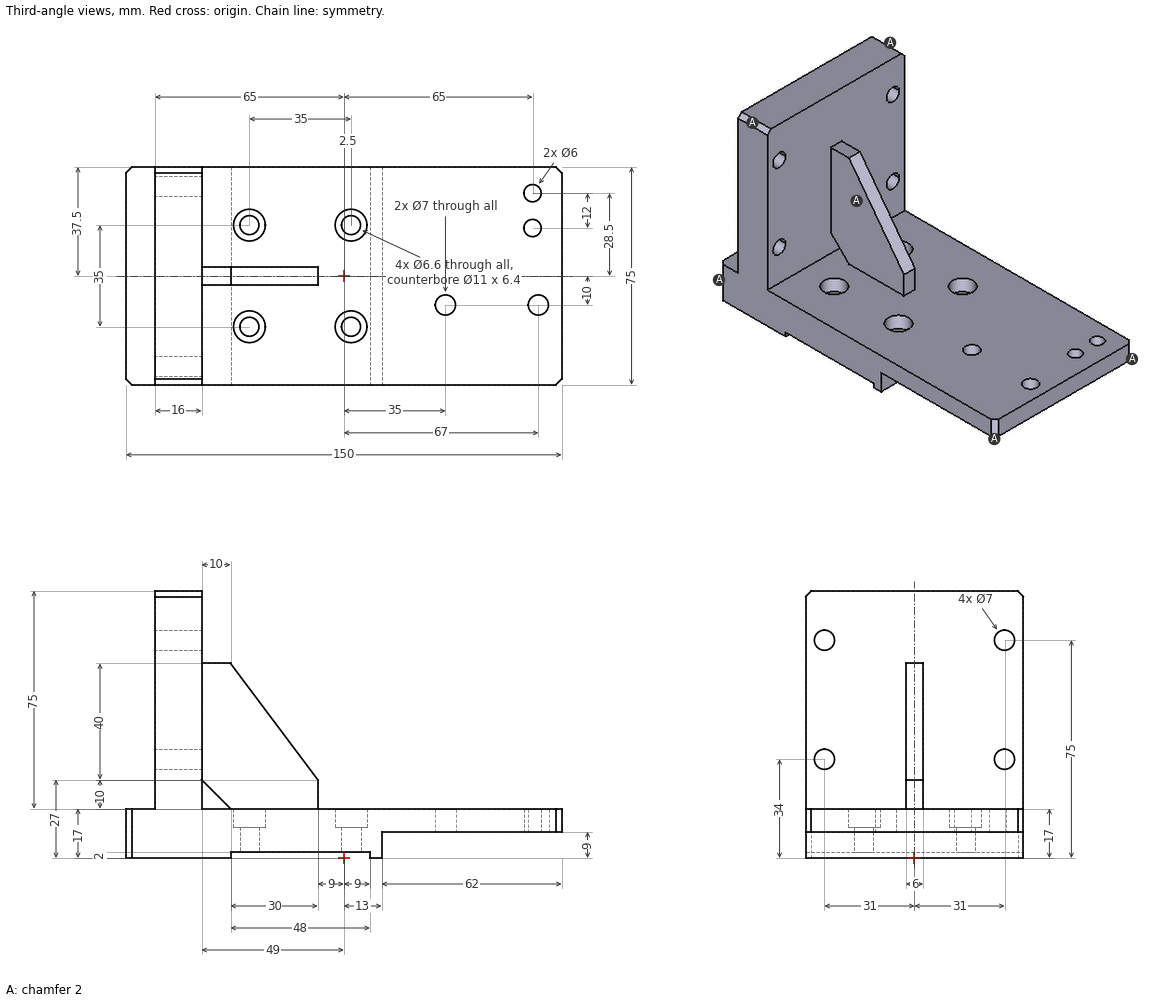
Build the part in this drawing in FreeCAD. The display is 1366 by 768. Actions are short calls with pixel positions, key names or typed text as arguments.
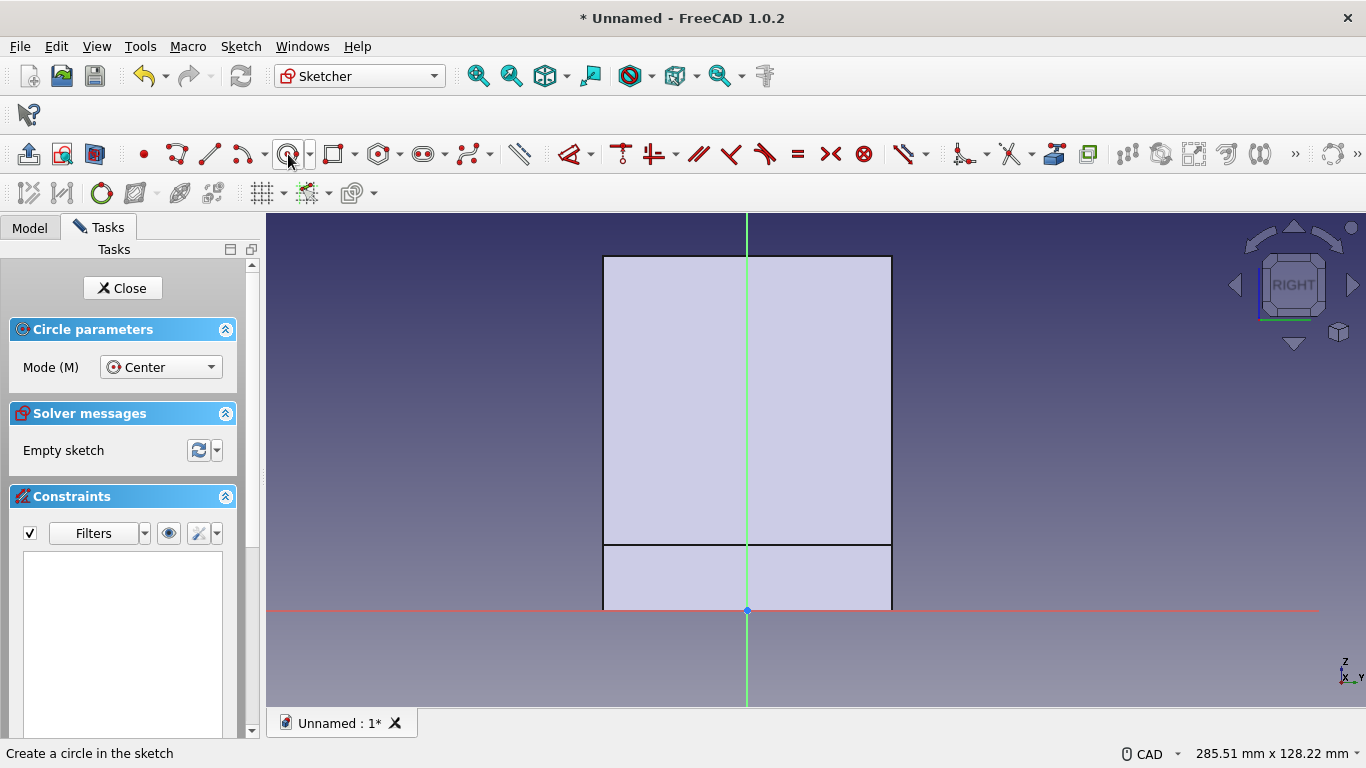
scroll(867, 322, up, 3)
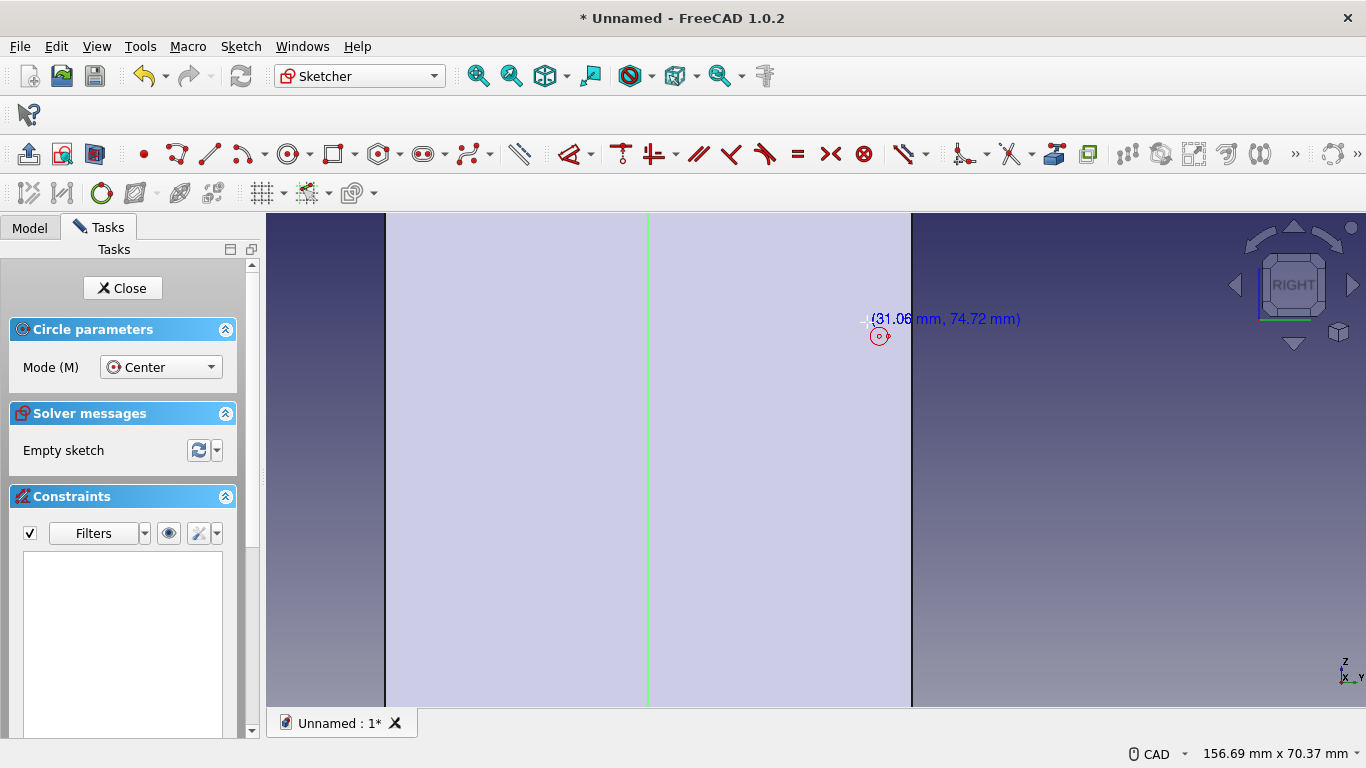
click(866, 322)
move(883, 304)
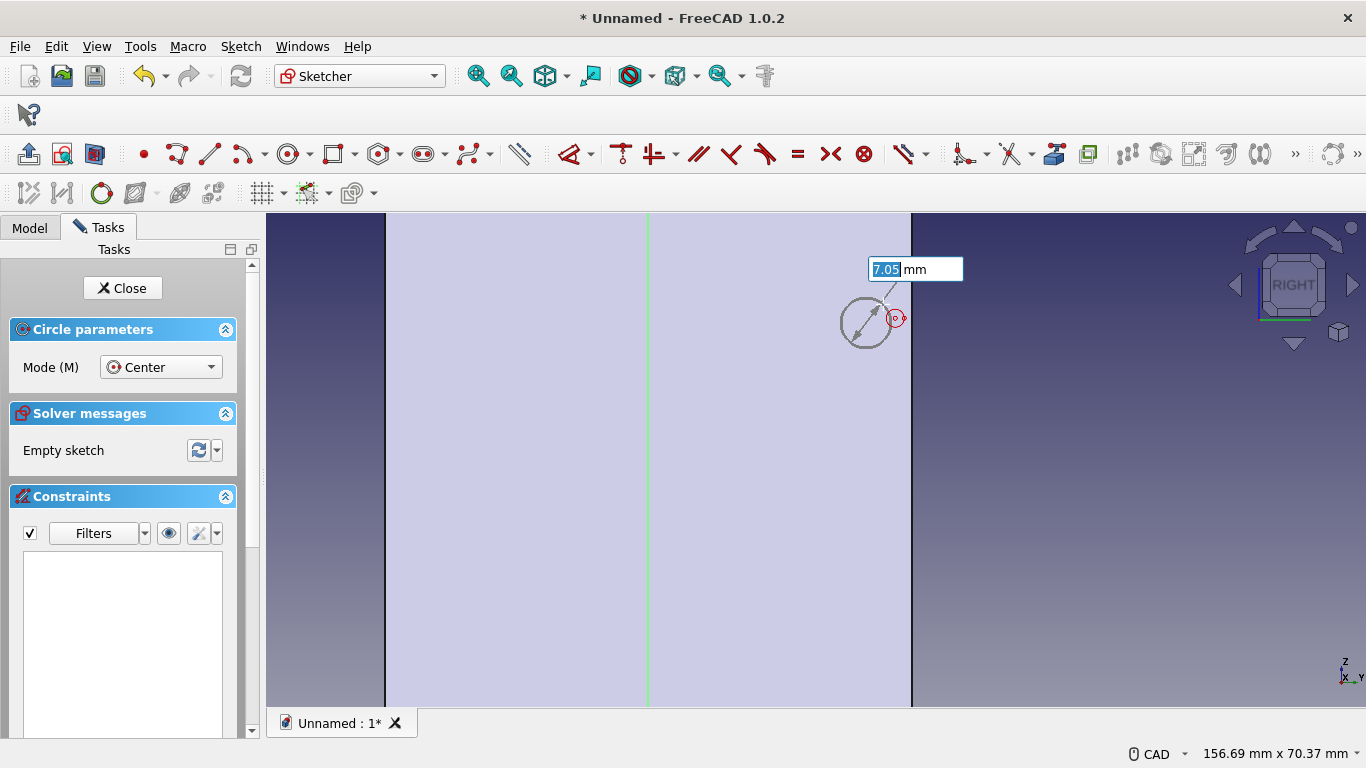
text(7)
key(Return)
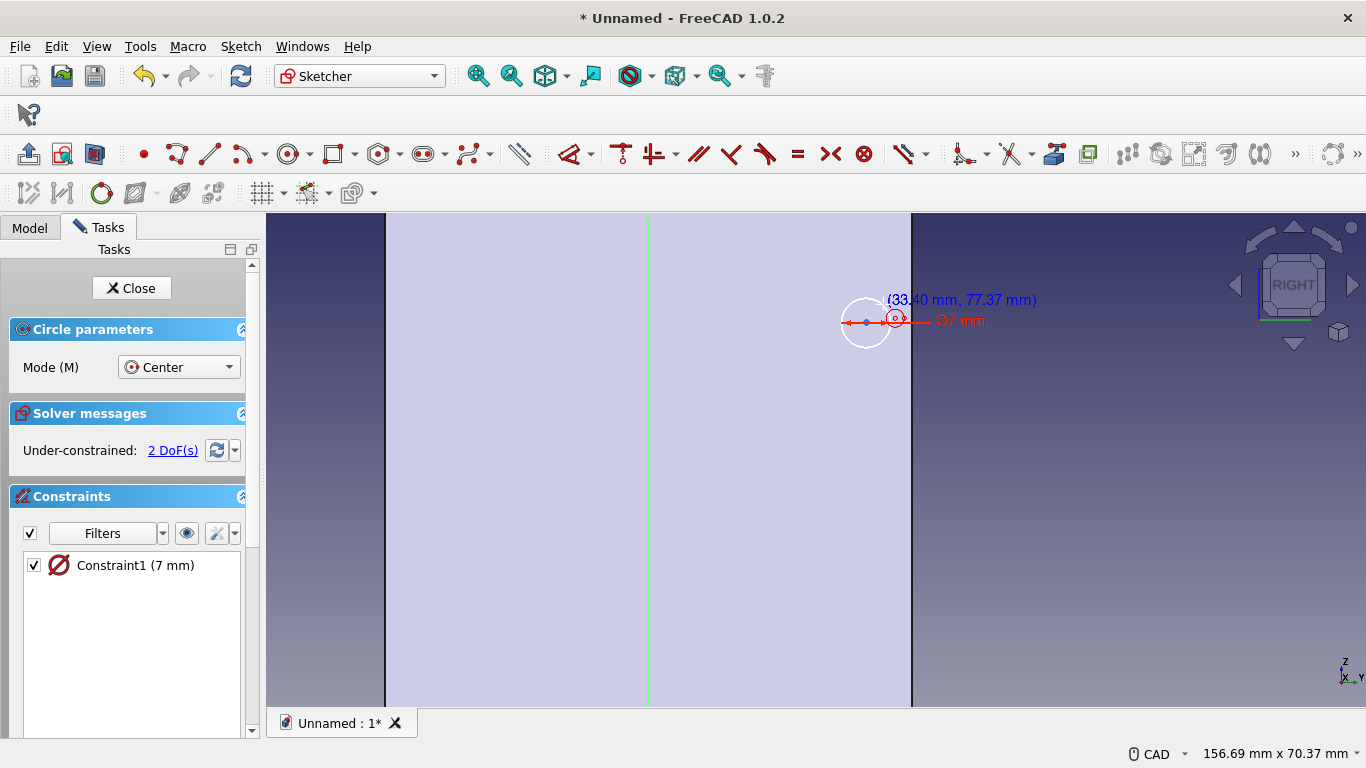
click(431, 322)
move(448, 304)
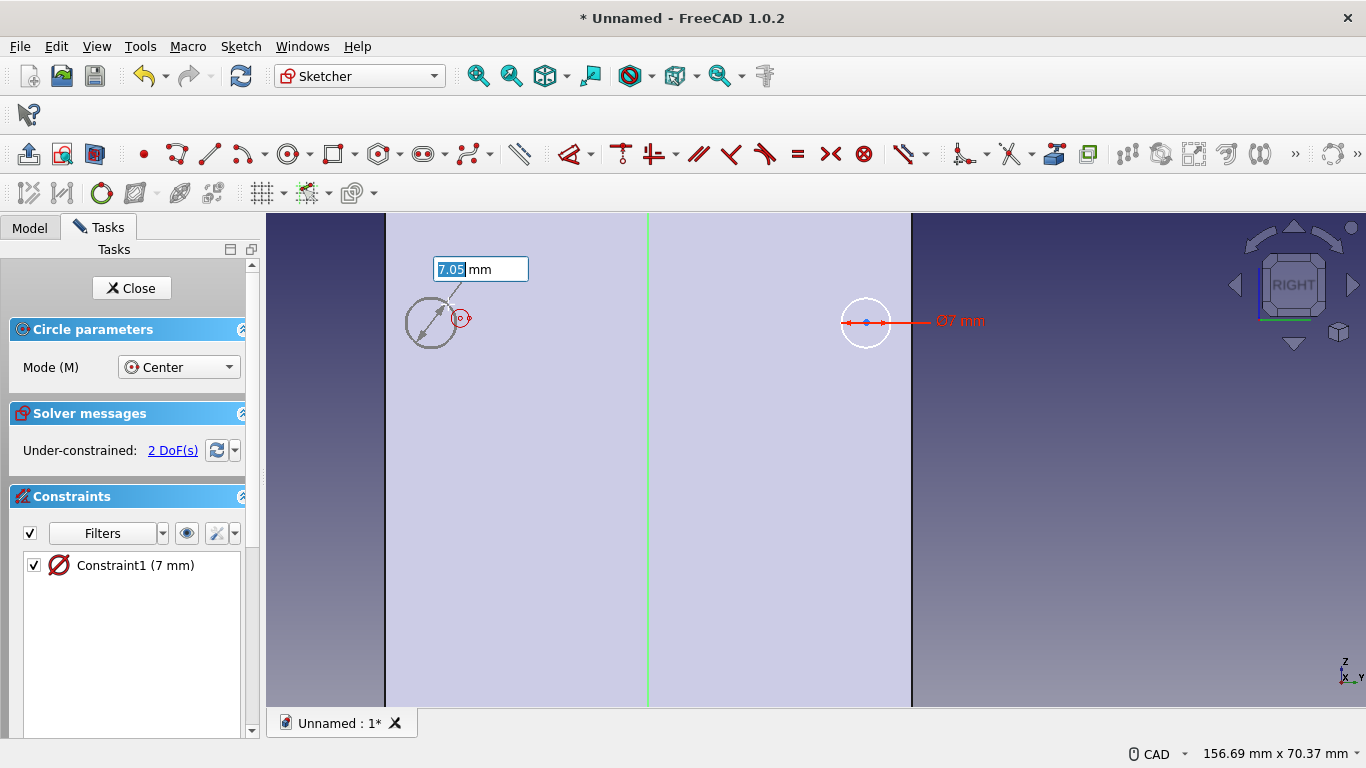
text(7)
key(Return)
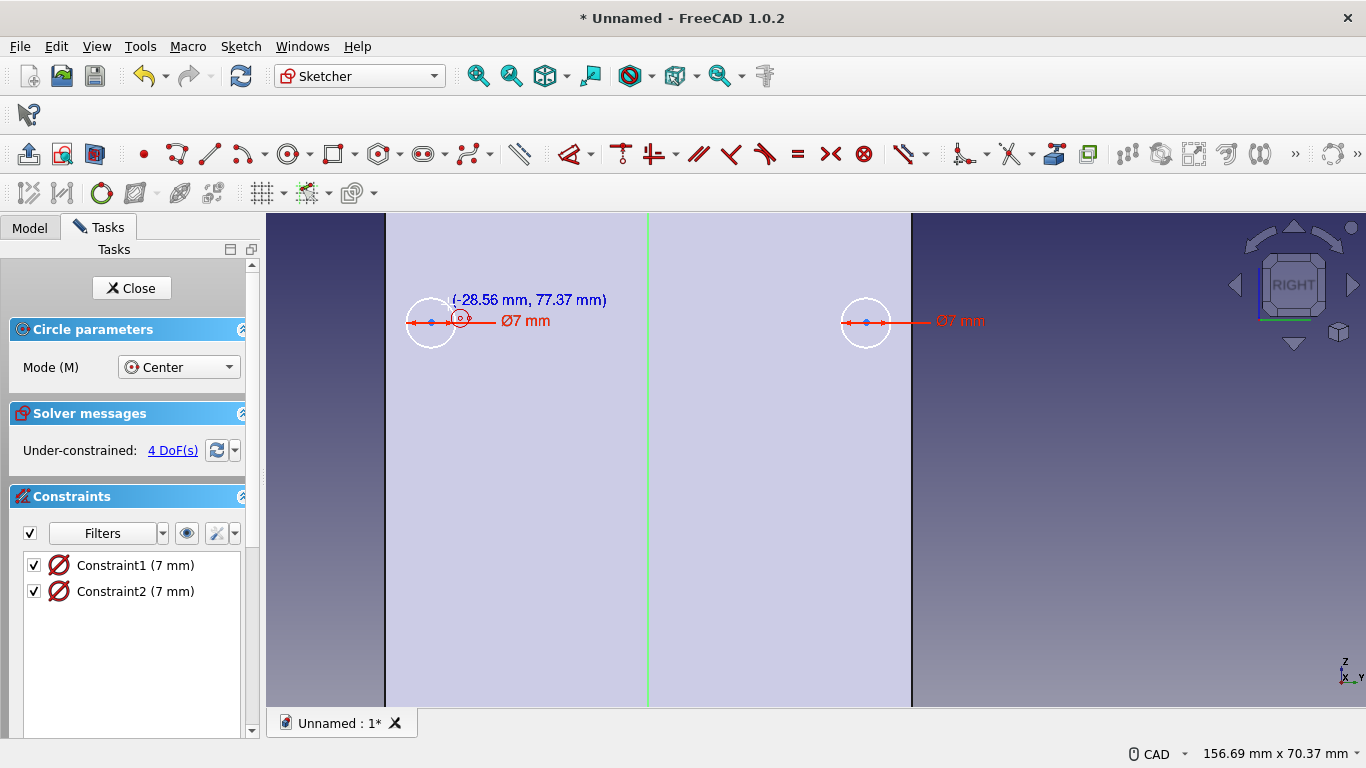
click(431, 609)
move(448, 592)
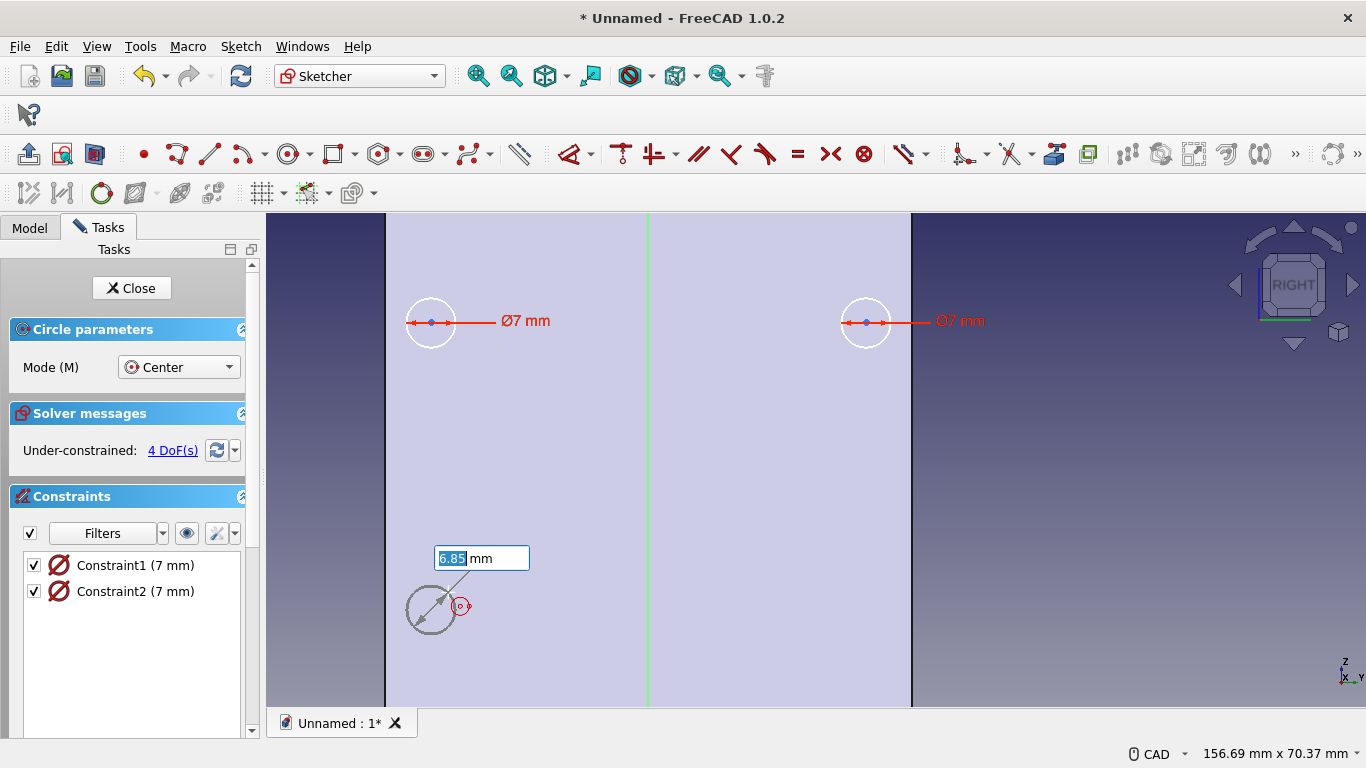
text(7)
key(Return)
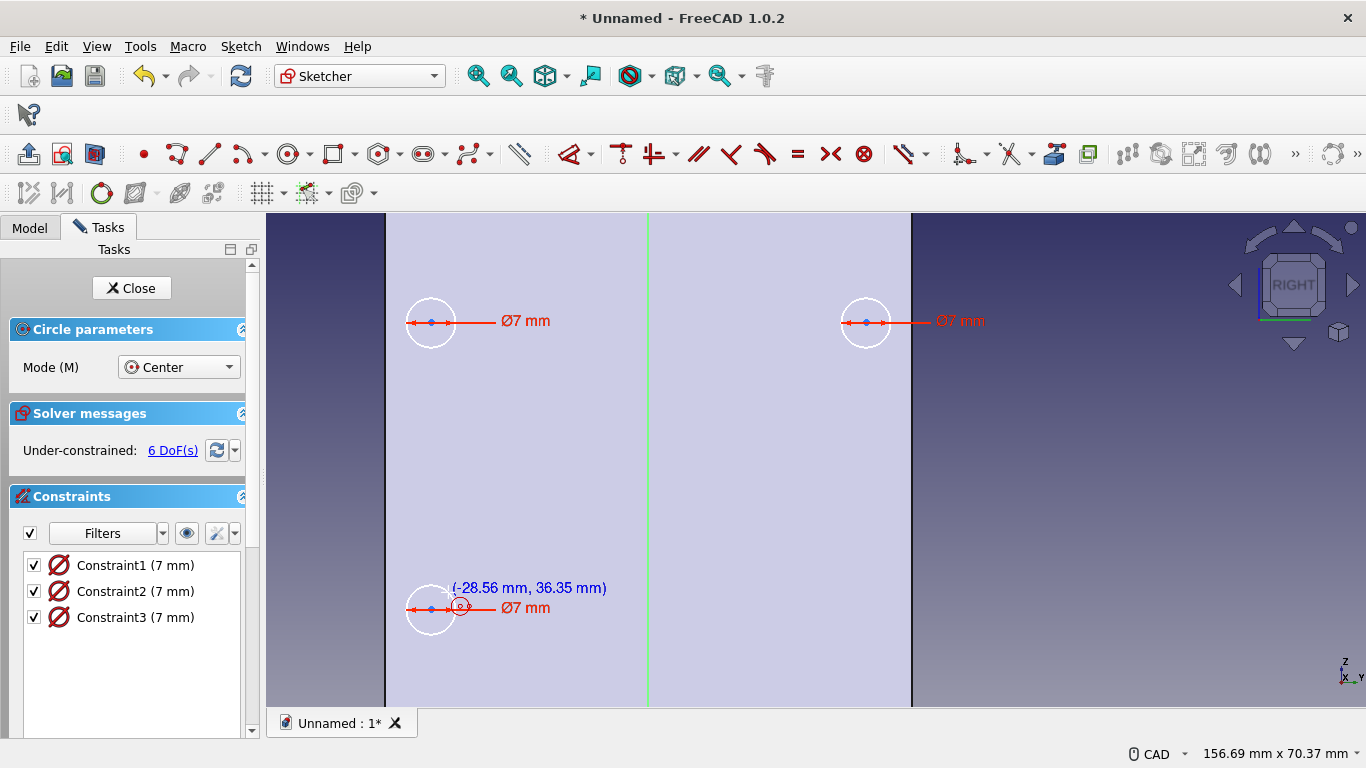
click(866, 609)
move(883, 592)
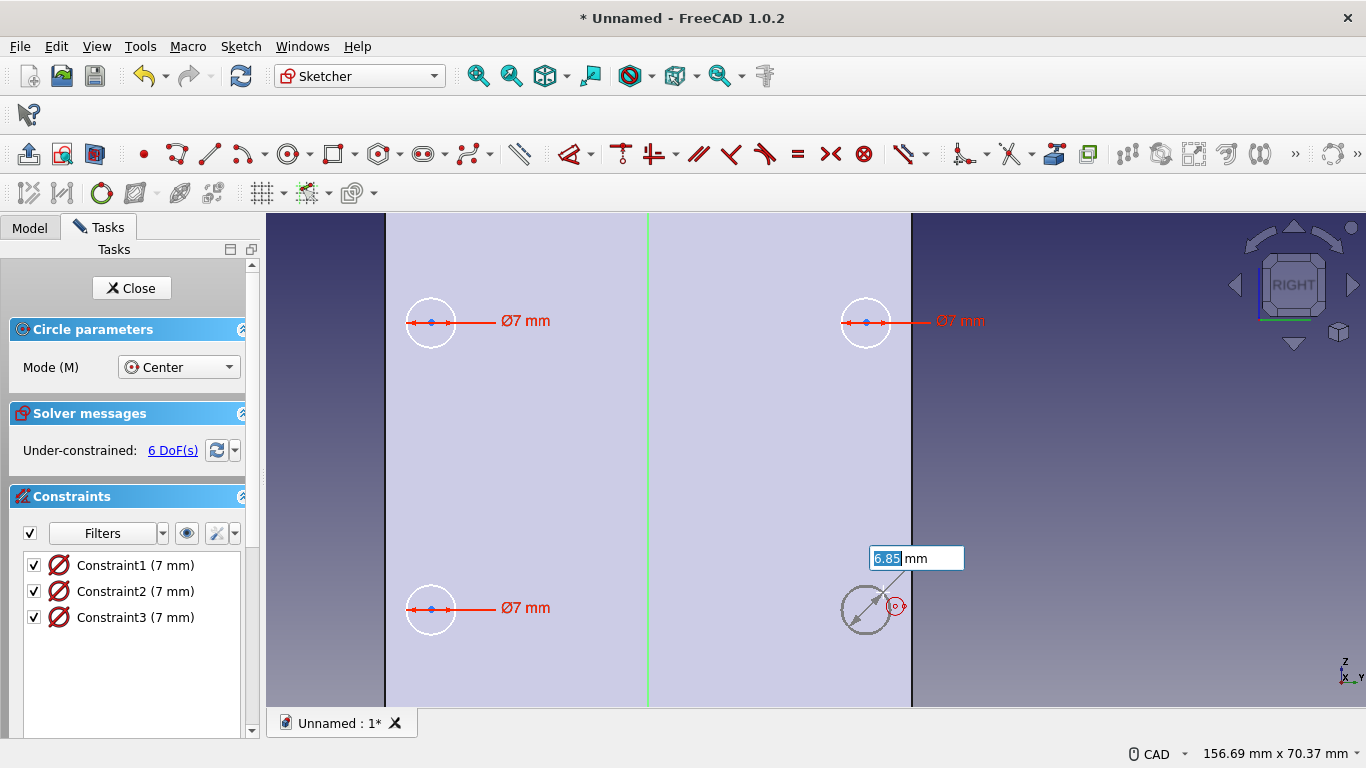
text(7)
key(Return)
key(Escape)